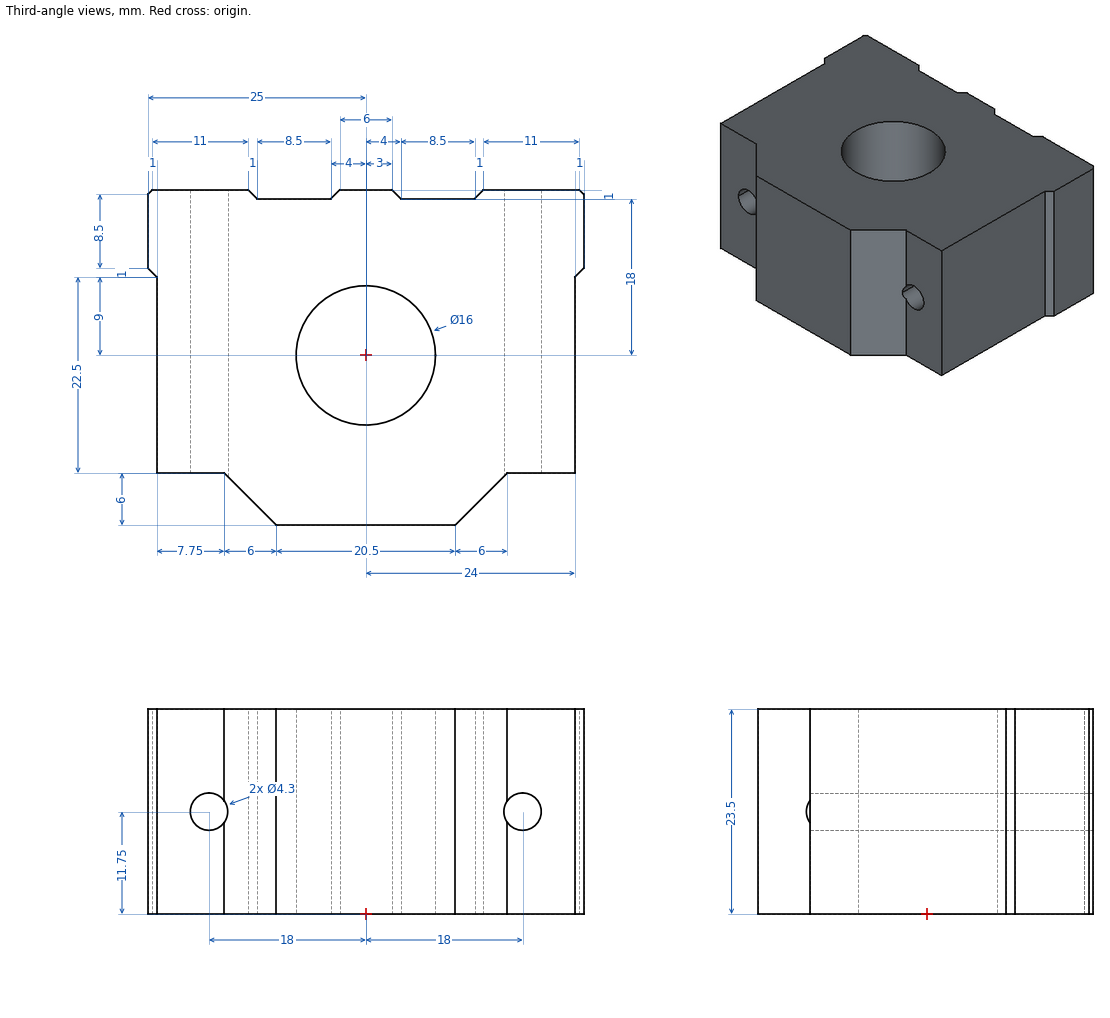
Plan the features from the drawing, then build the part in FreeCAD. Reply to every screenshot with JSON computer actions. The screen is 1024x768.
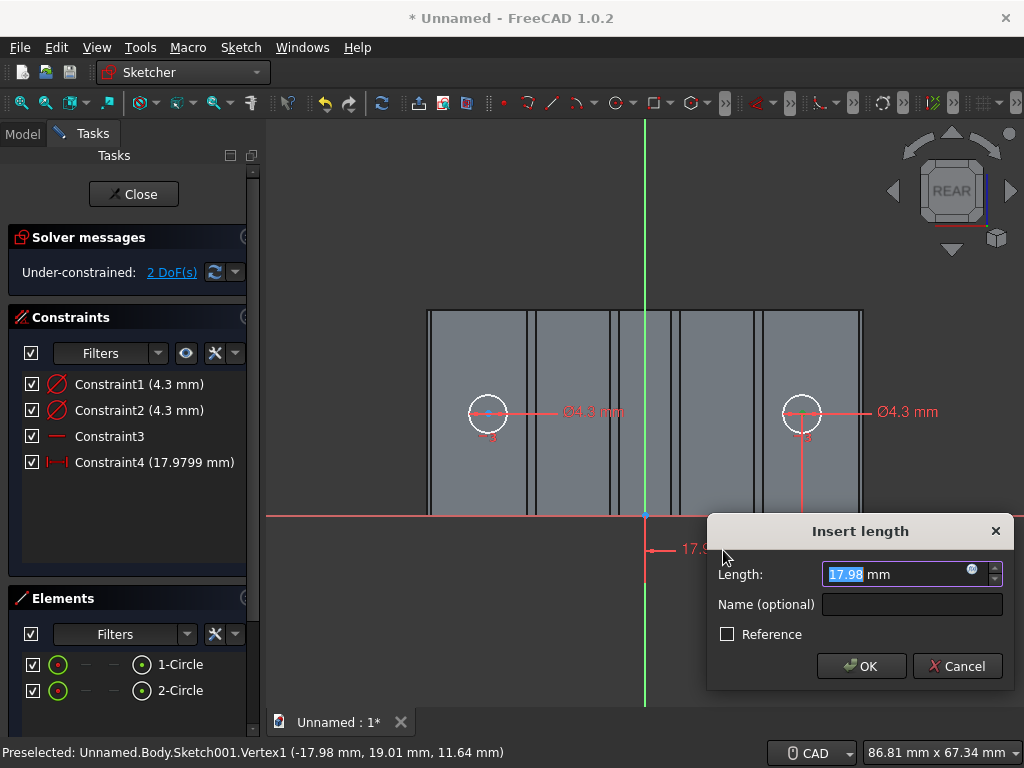
{"action": "type", "text": "18"}
{"action": "key", "text": "Return"}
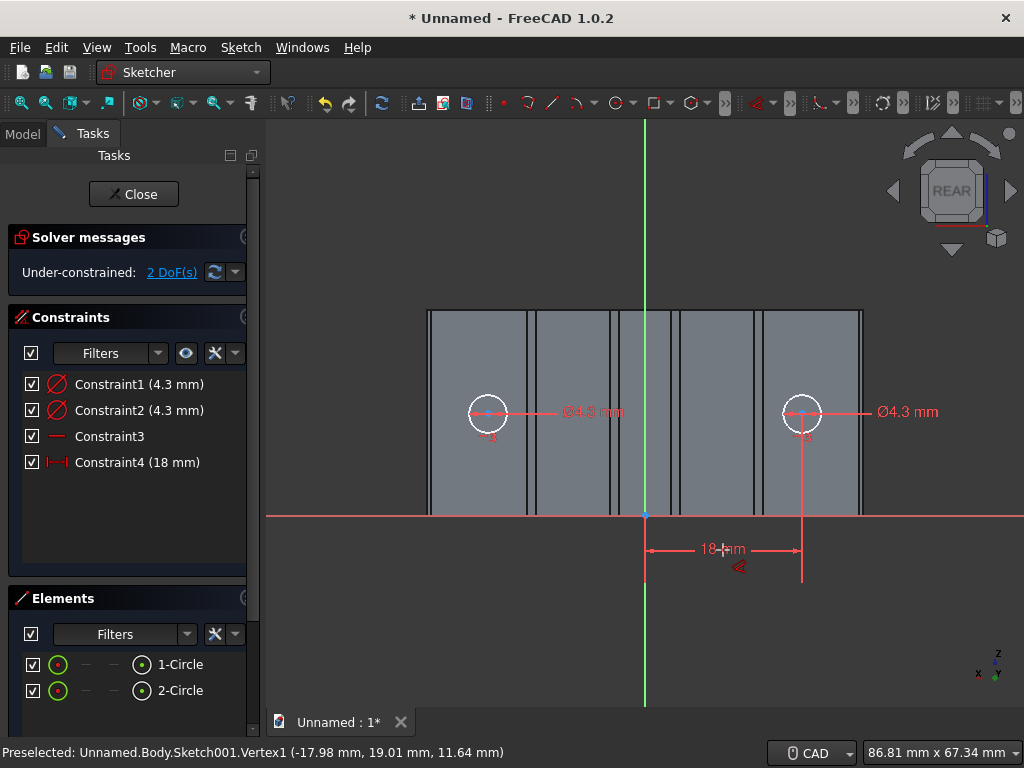
{"action": "left_click", "coordinate": [488, 414]}
{"action": "left_click", "coordinate": [566, 550]}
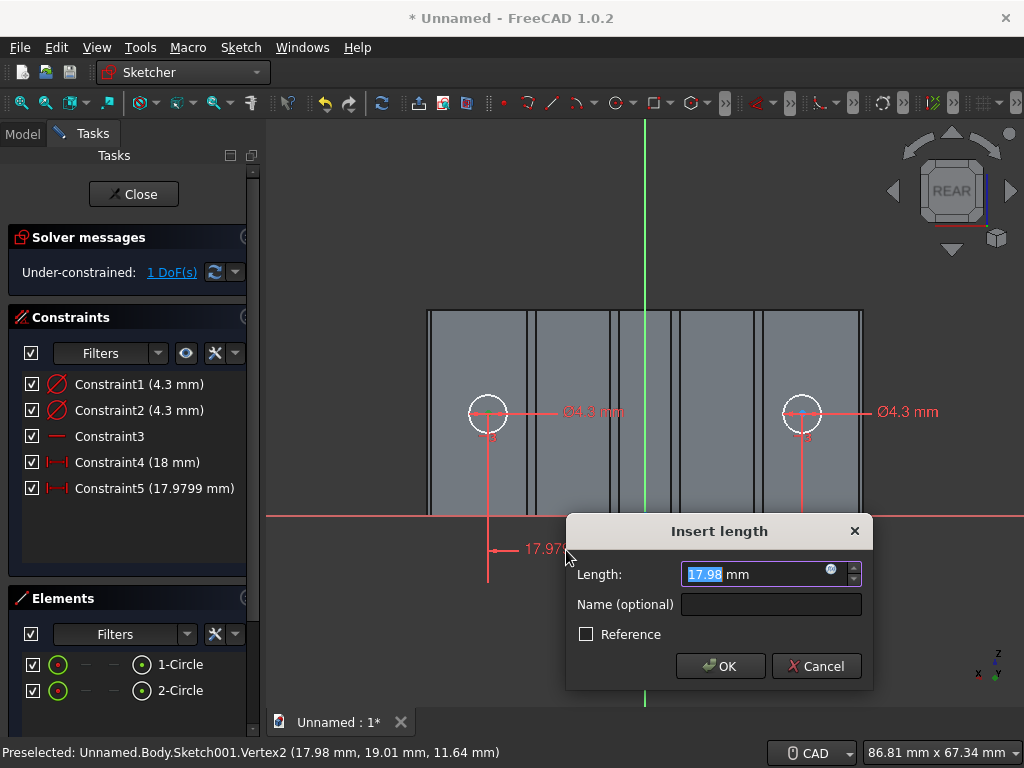
{"action": "type", "text": "18"}
{"action": "key", "text": "Return"}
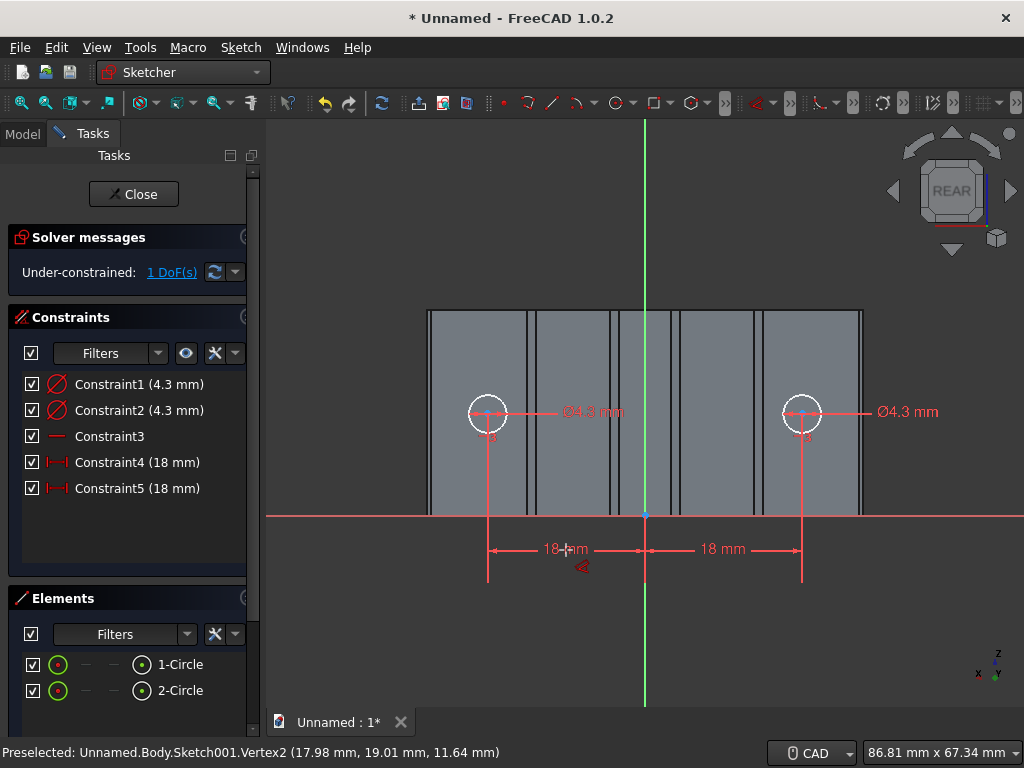
{"action": "left_click", "coordinate": [802, 414]}
{"action": "left_click", "coordinate": [836, 465]}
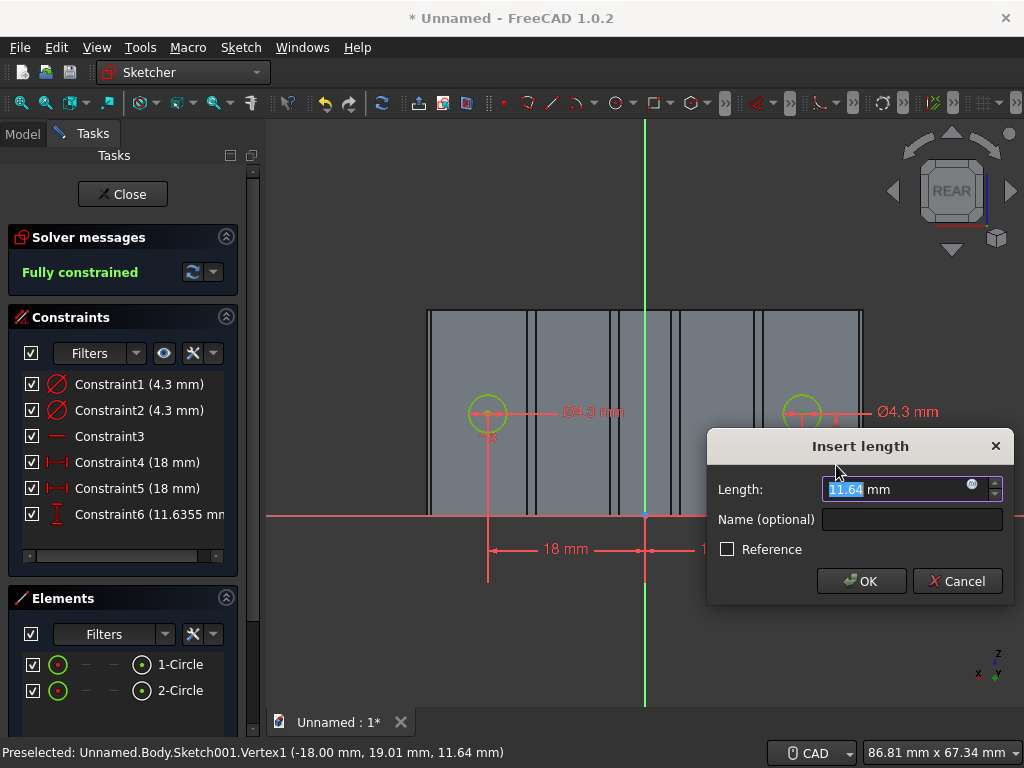
{"action": "type", "text": "11.75"}
{"action": "key", "text": "Return"}
{"action": "key", "text": "Escape"}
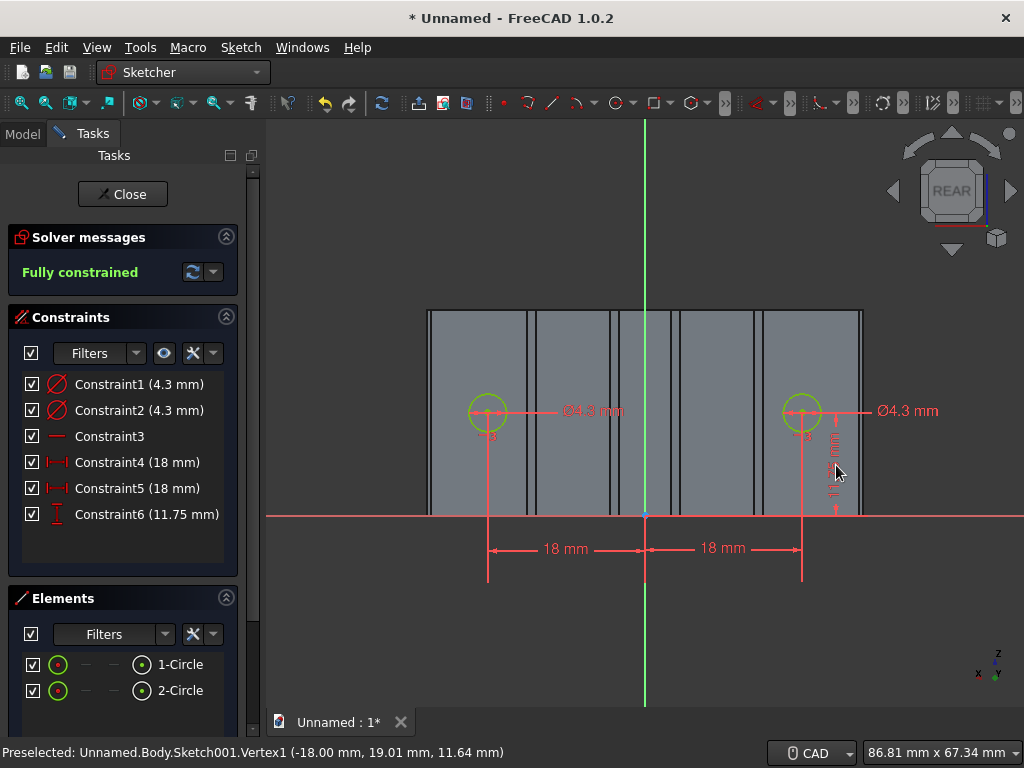
{"action": "left_click", "coordinate": [123, 194]}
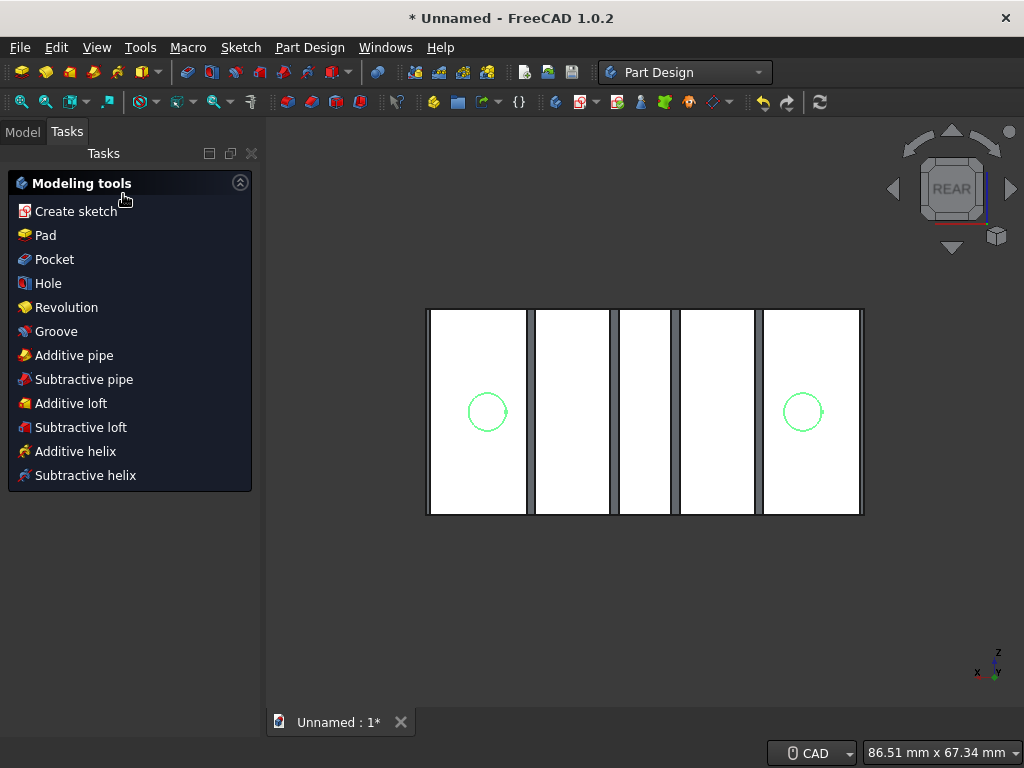
{"action": "left_click", "coordinate": [188, 72]}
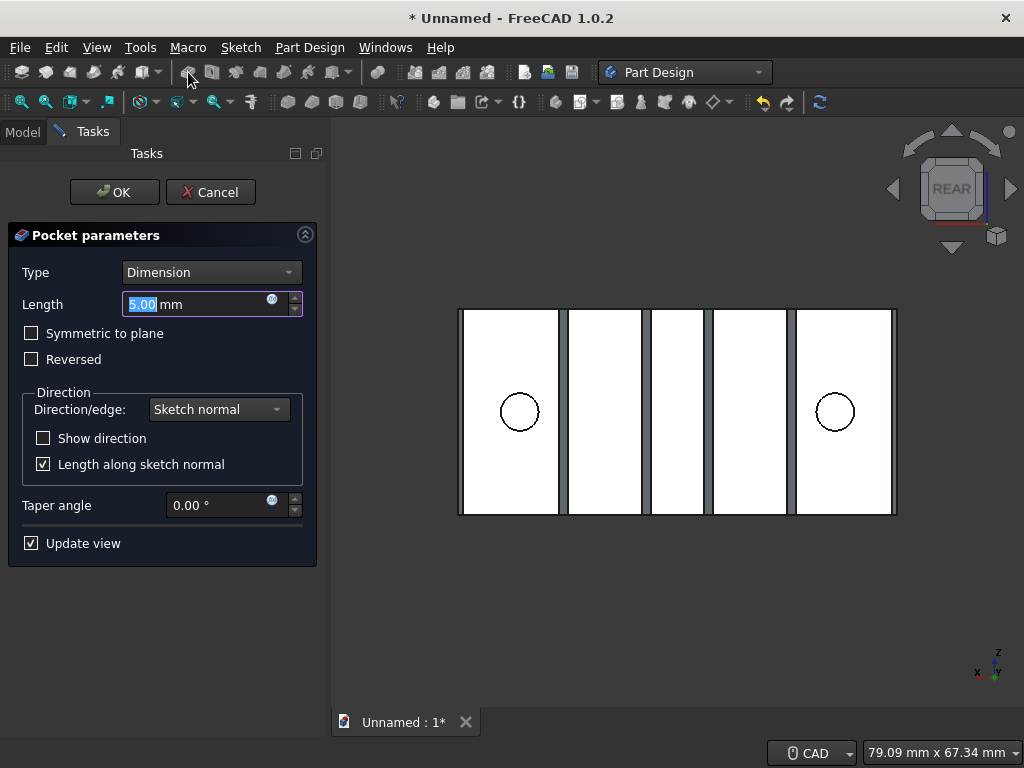
{"action": "left_click", "coordinate": [212, 272]}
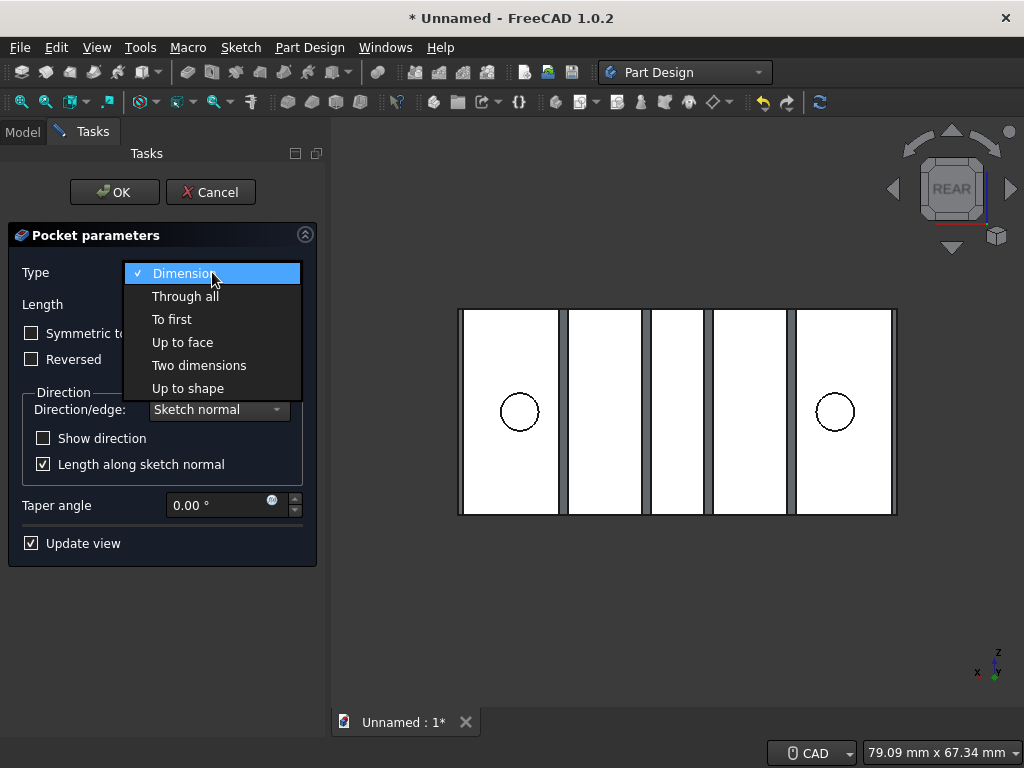
{"action": "left_click", "coordinate": [212, 296]}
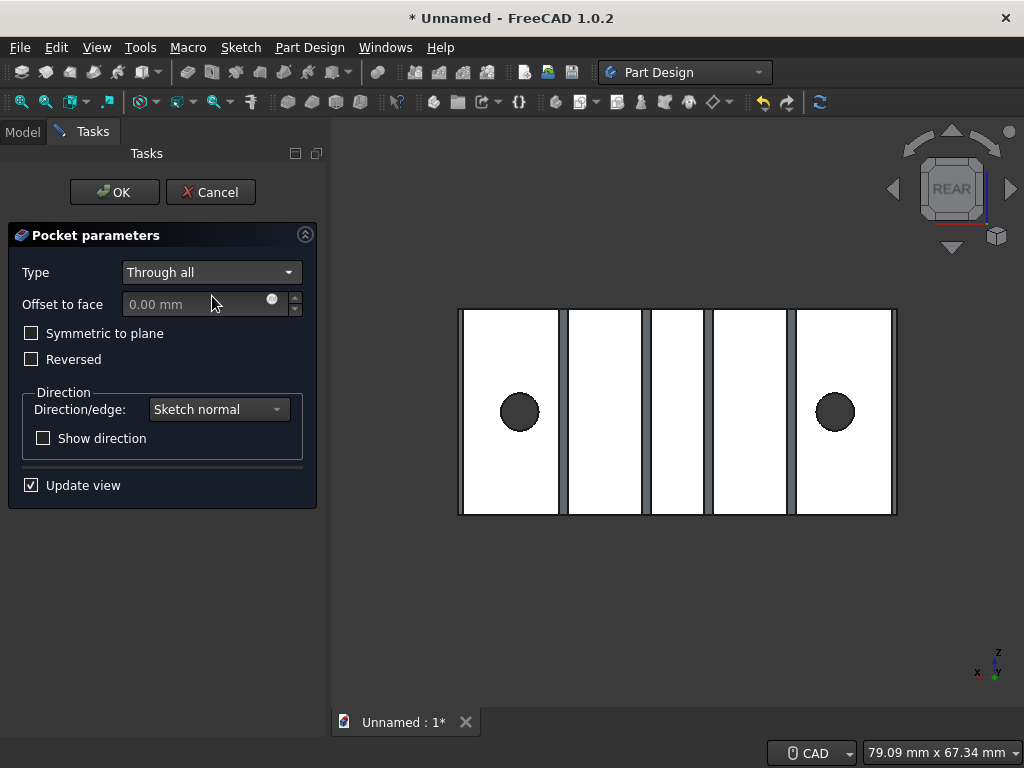
{"action": "left_click", "coordinate": [115, 192]}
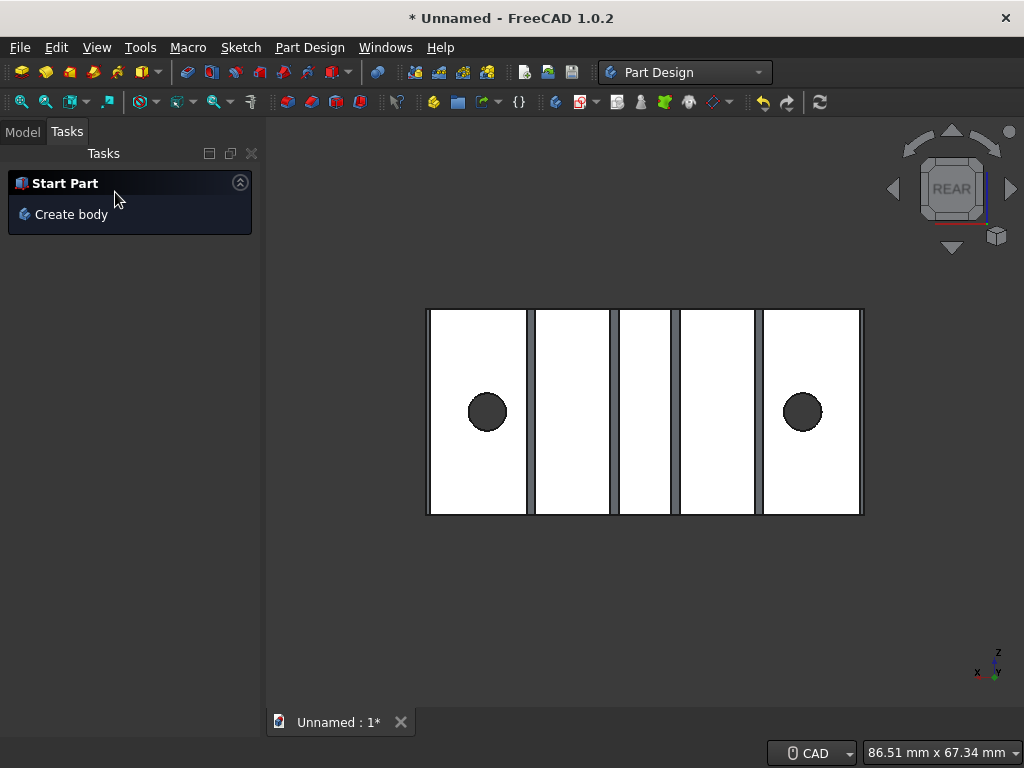
{"action": "key", "text": "0"}